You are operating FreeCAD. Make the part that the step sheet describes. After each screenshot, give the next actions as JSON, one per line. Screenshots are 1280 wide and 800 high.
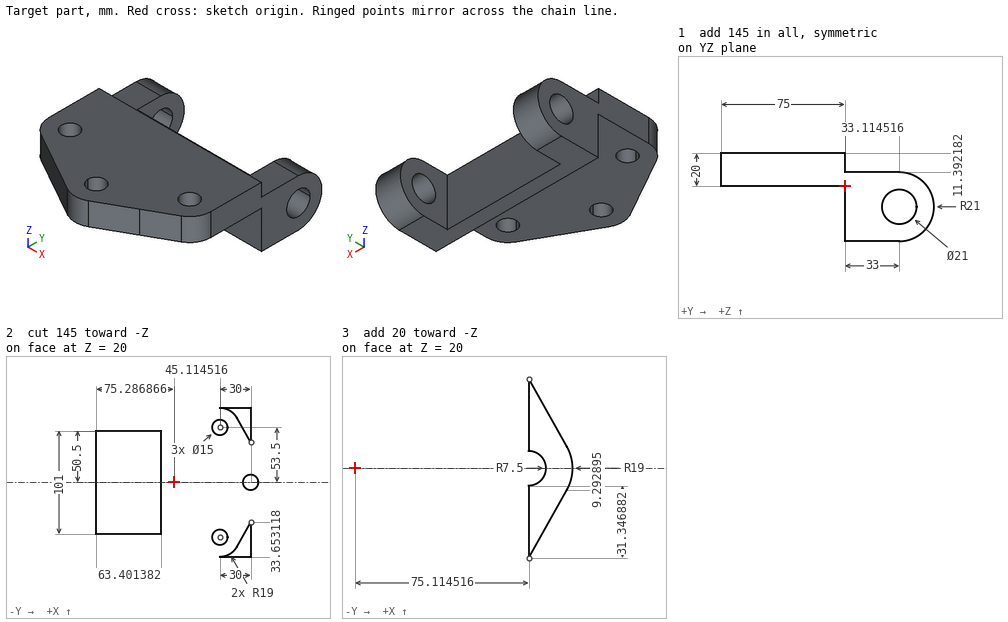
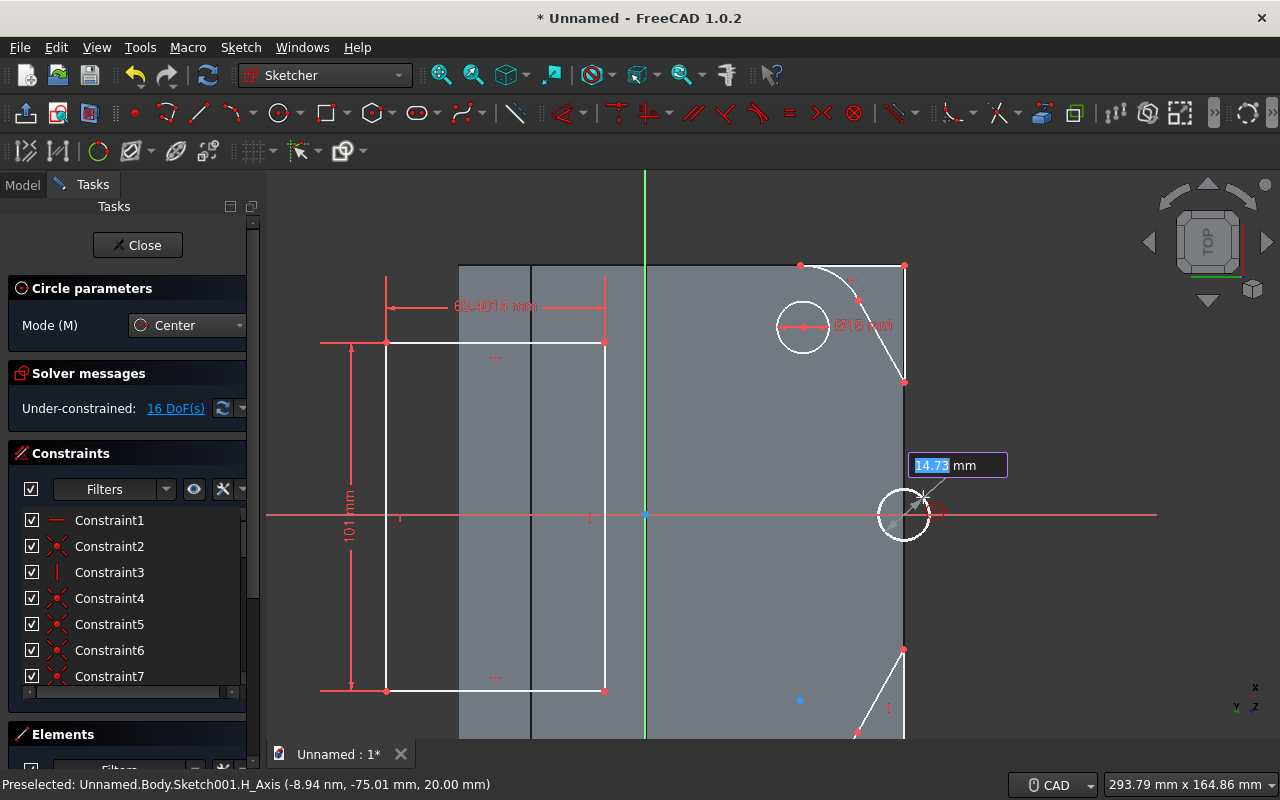
{"action": "type", "text": "15"}
{"action": "key", "text": "Return"}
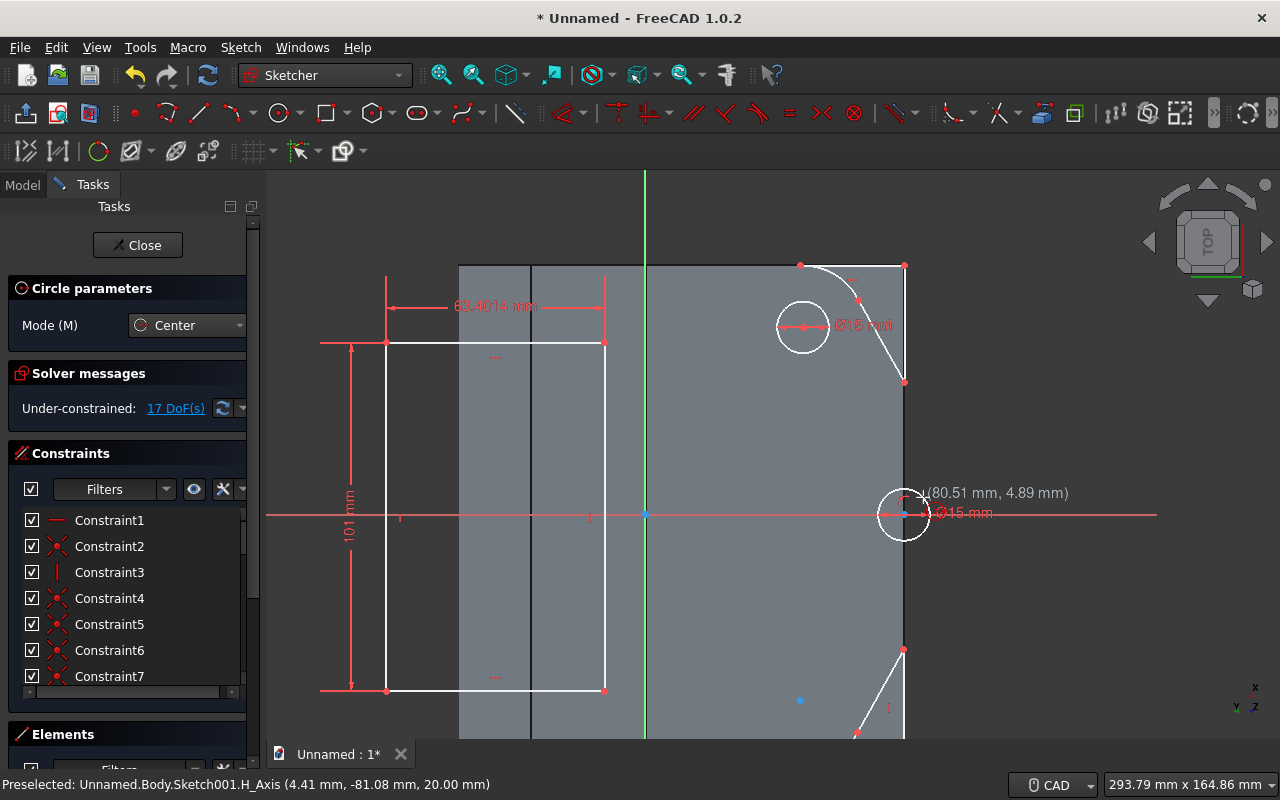
{"action": "left_click", "coordinate": [801, 700]}
{"action": "mouse_move", "coordinate": [819, 681]}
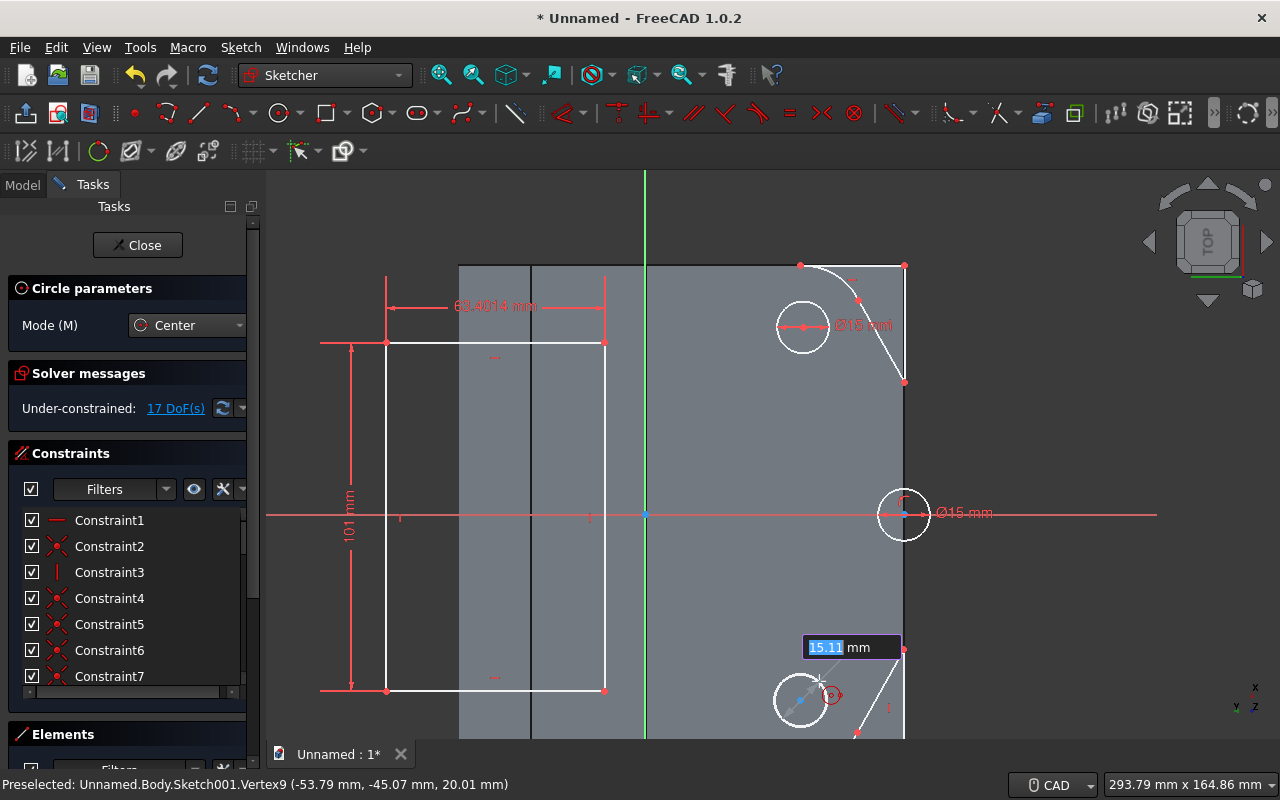
{"action": "type", "text": "15"}
{"action": "key", "text": "Return"}
{"action": "key", "text": "Escape"}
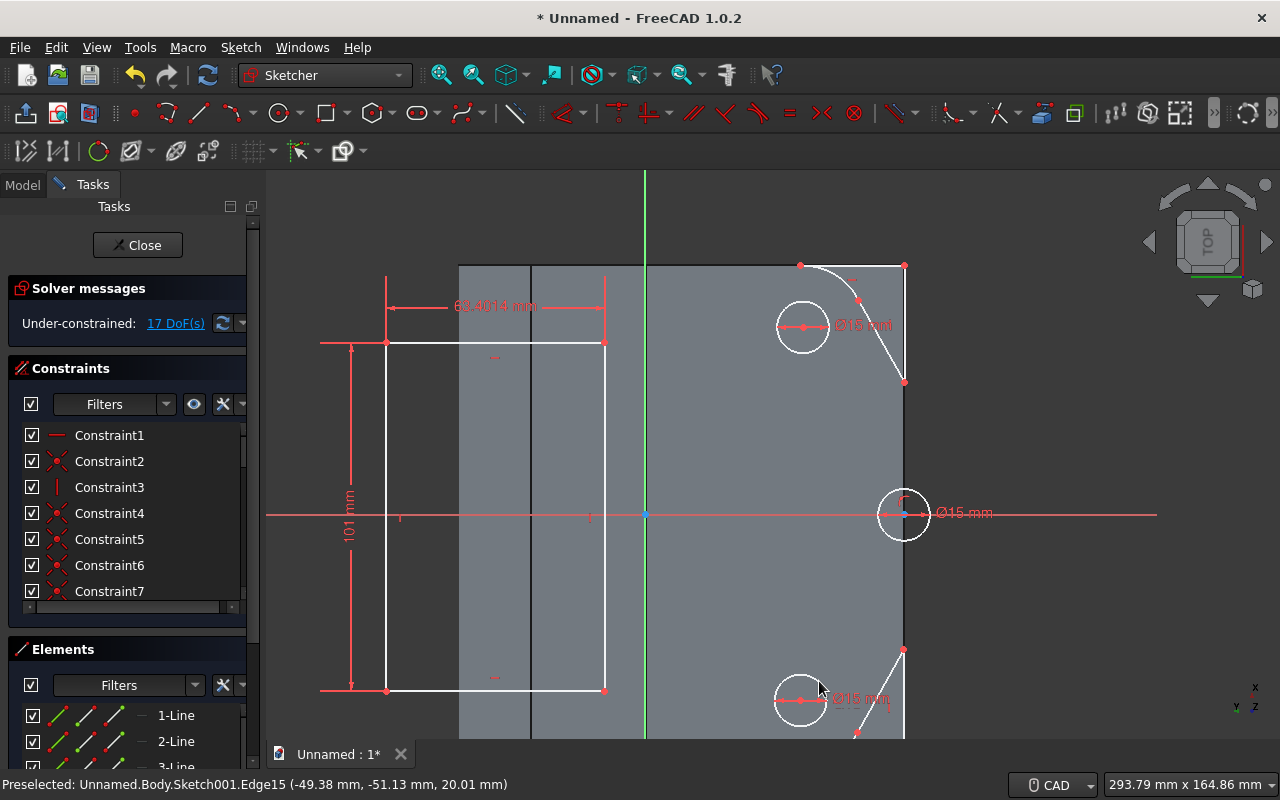
{"action": "scroll", "coordinate": [800, 332], "scroll_direction": "down", "scroll_amount": 2}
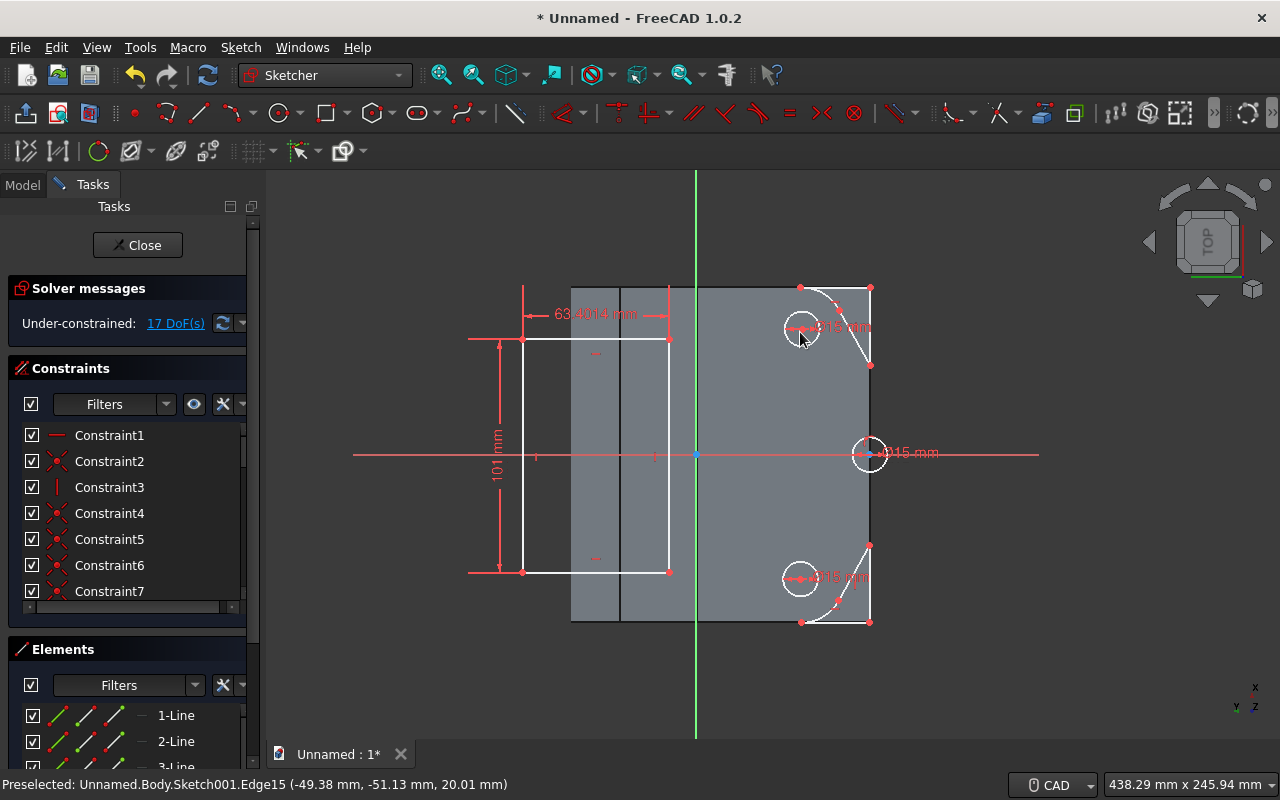
{"action": "left_click", "coordinate": [849, 623]}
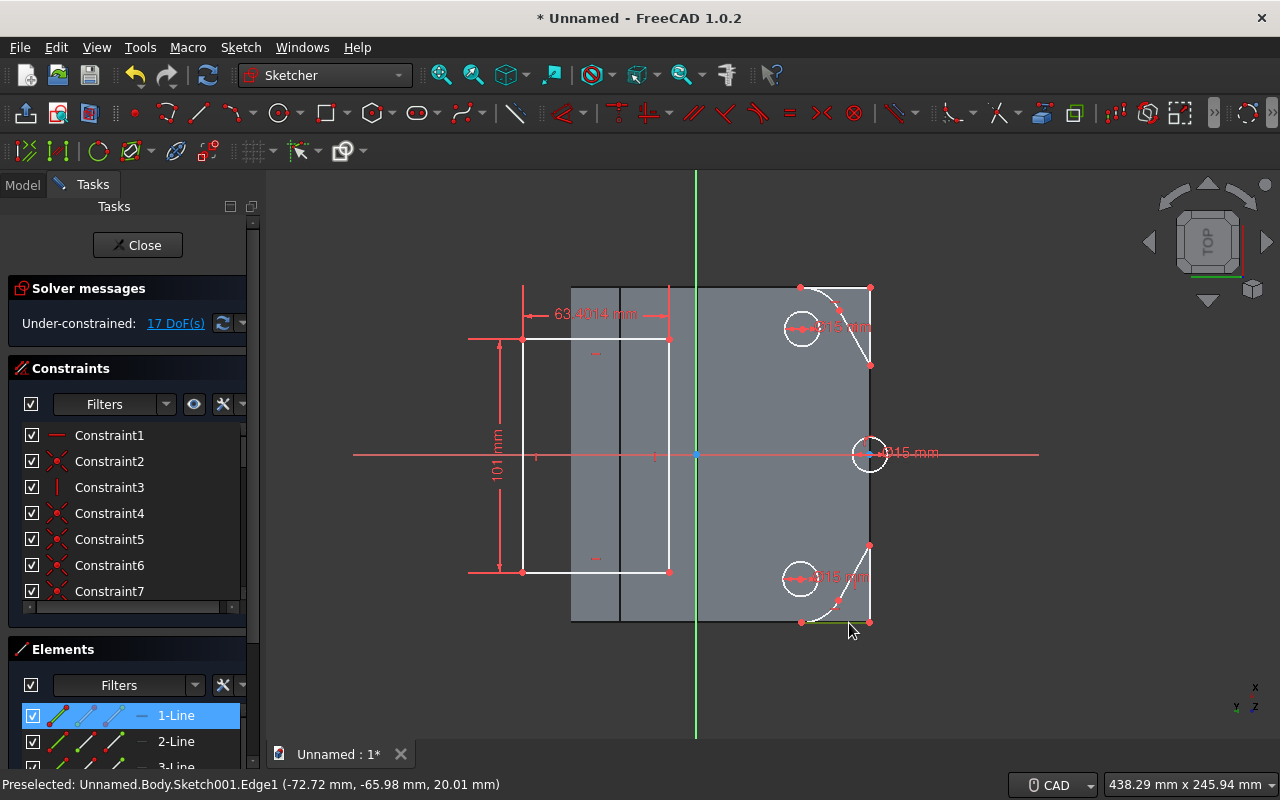
{"action": "scroll", "coordinate": [830, 611], "scroll_direction": "up", "scroll_amount": 4}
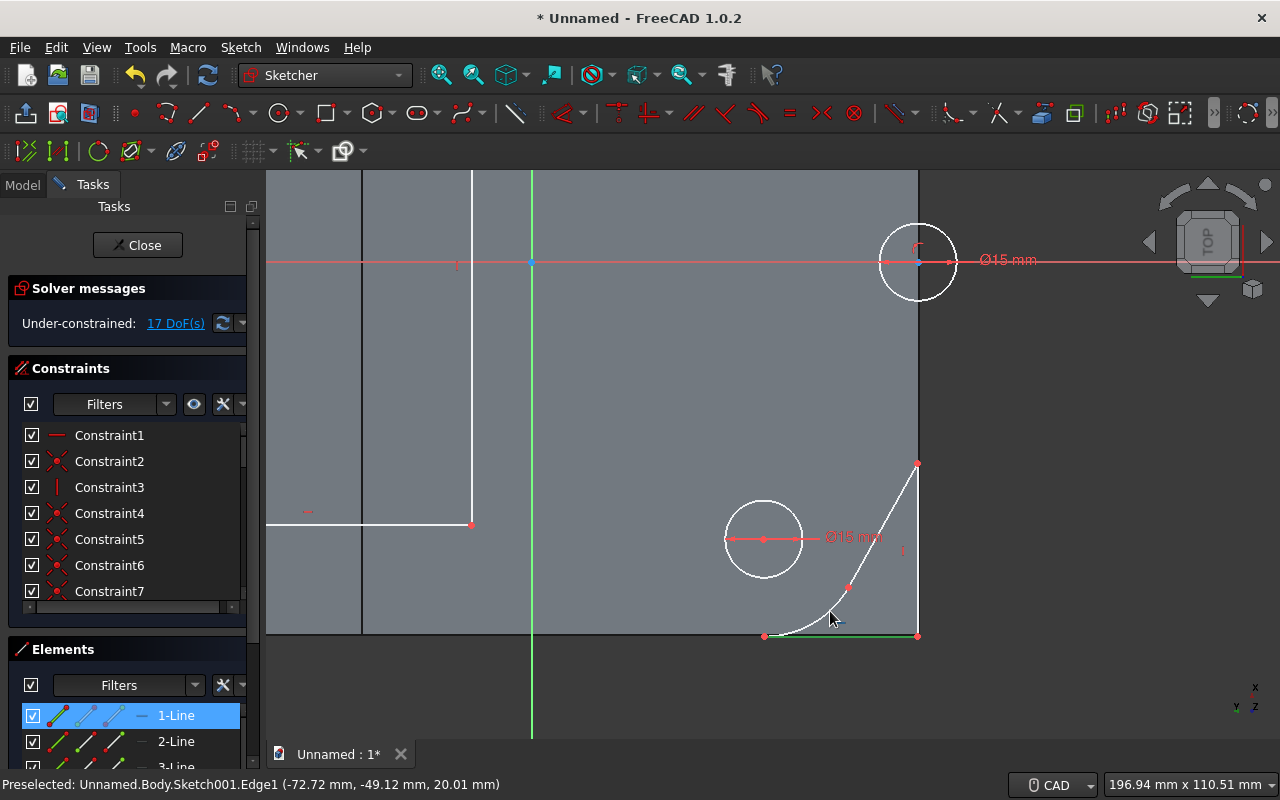
{"action": "left_click", "coordinate": [830, 611]}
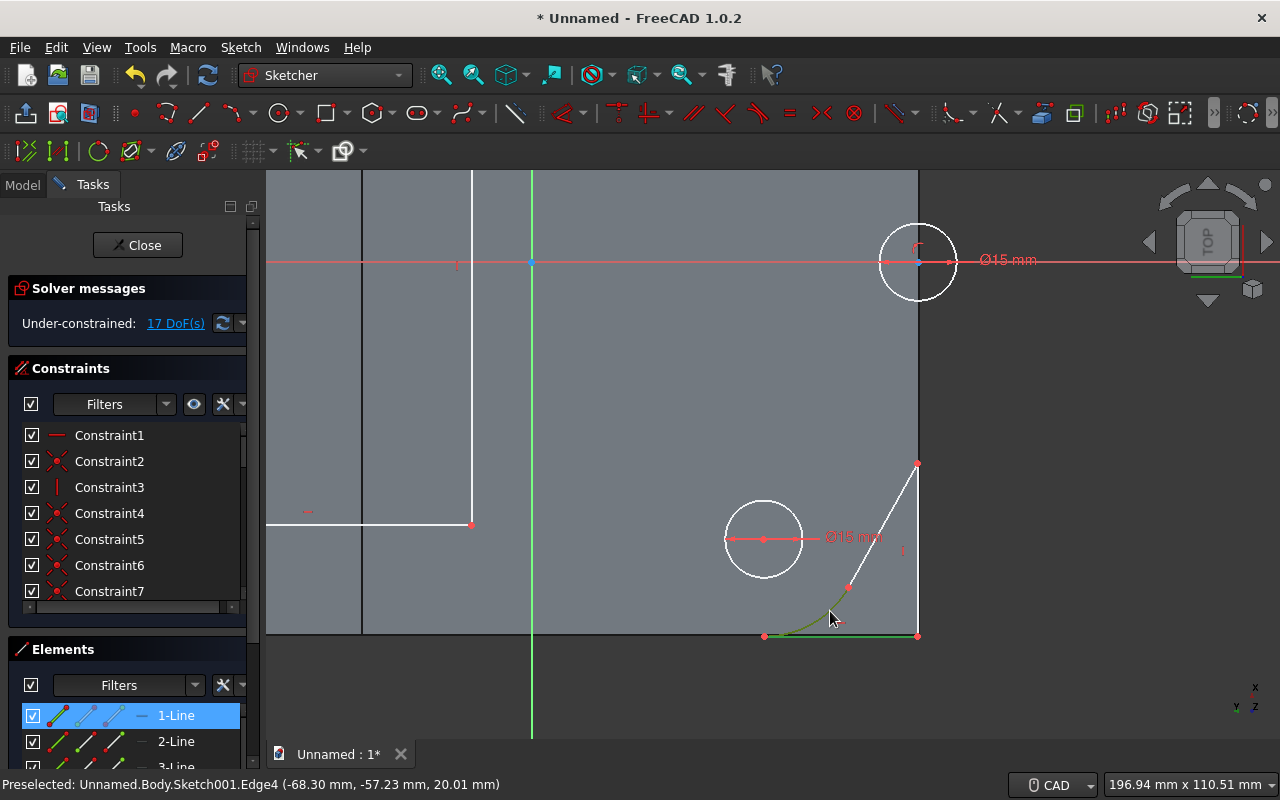
{"action": "left_click", "coordinate": [758, 114]}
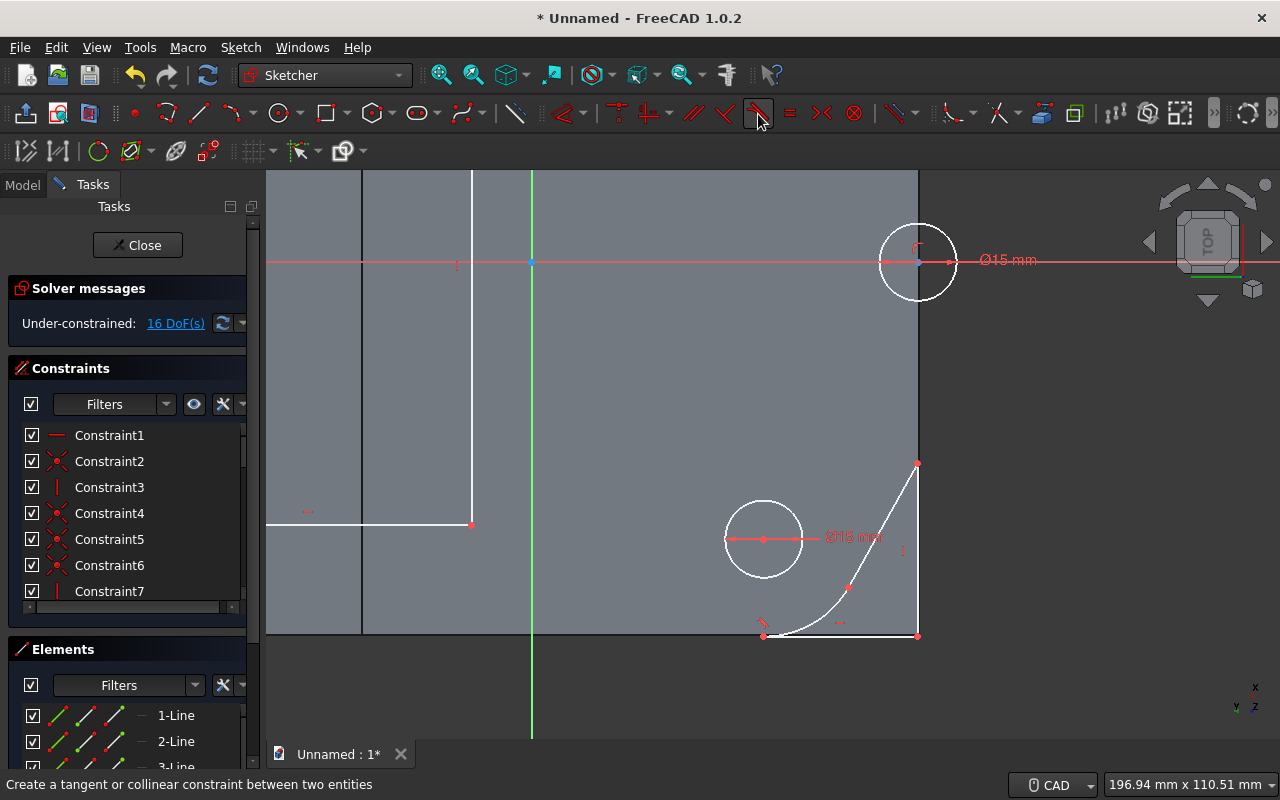
{"action": "left_click", "coordinate": [897, 501]}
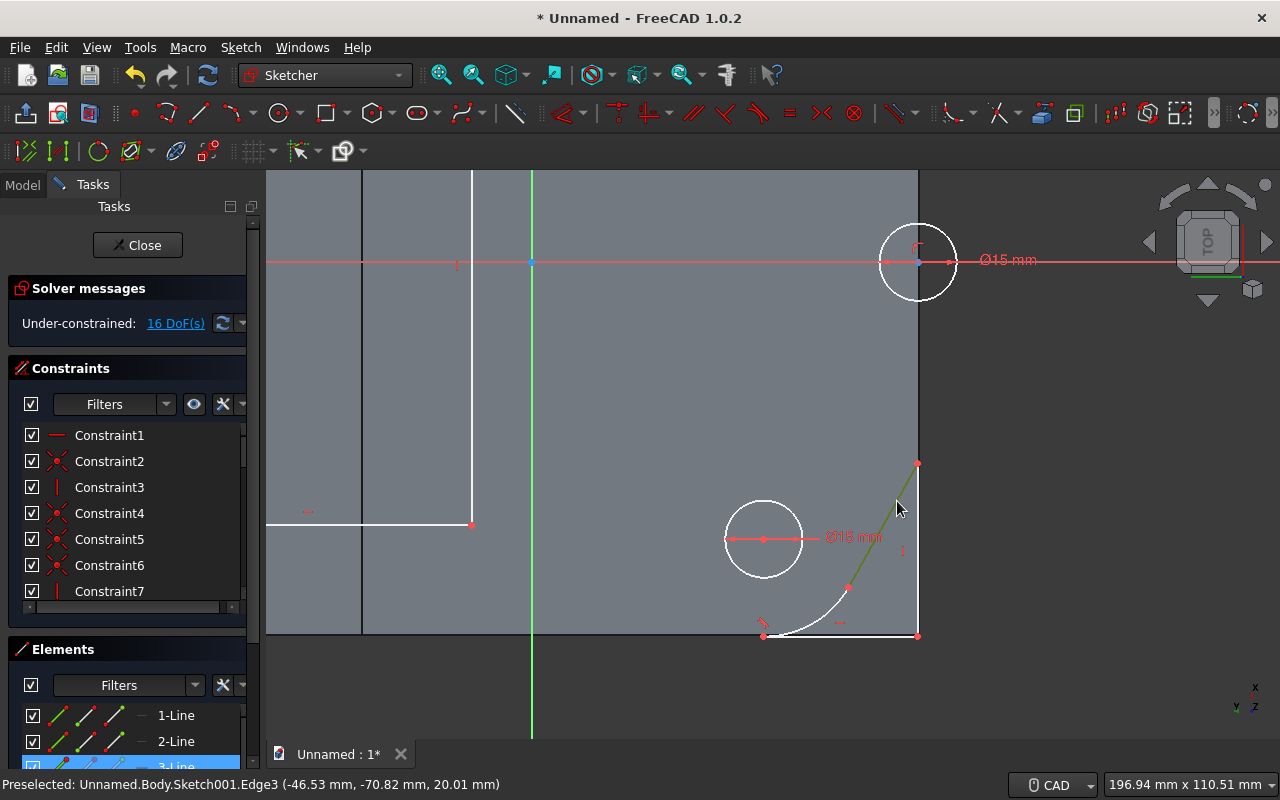
{"action": "left_click", "coordinate": [829, 611]}